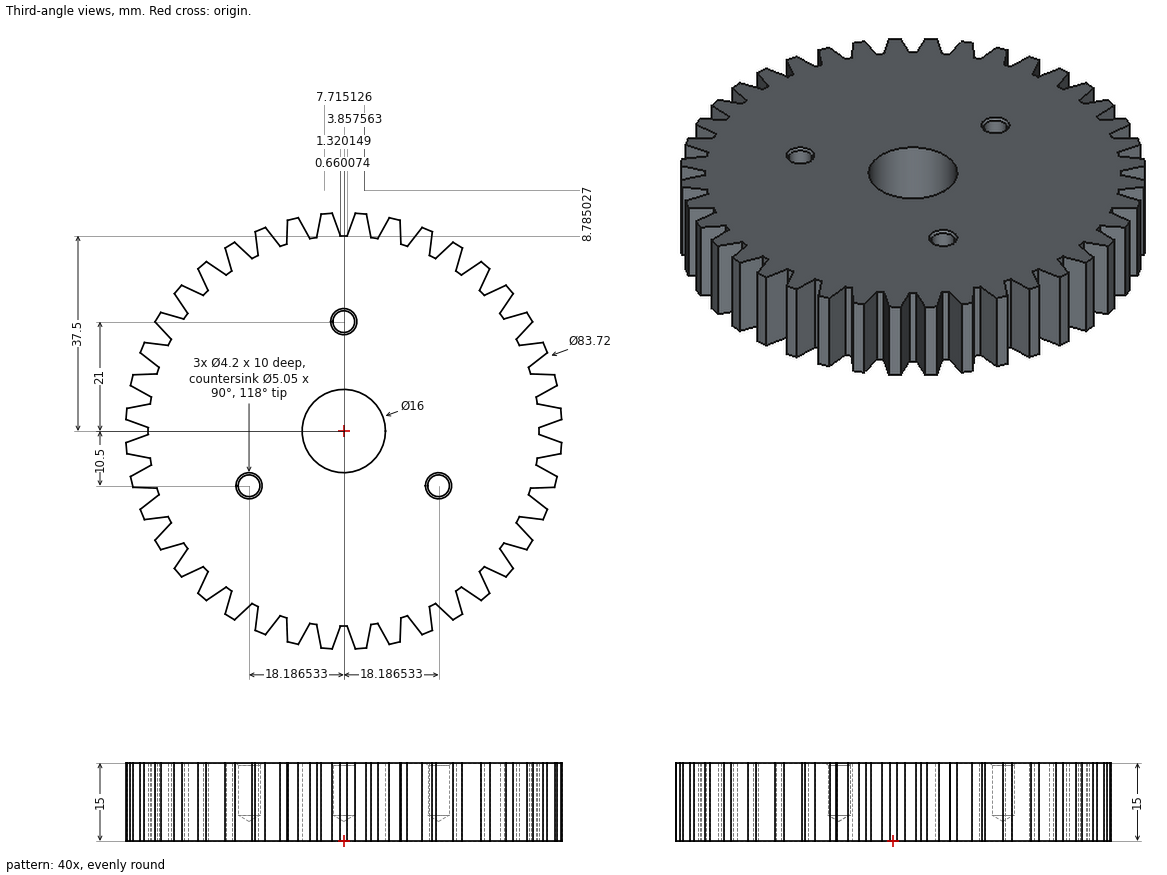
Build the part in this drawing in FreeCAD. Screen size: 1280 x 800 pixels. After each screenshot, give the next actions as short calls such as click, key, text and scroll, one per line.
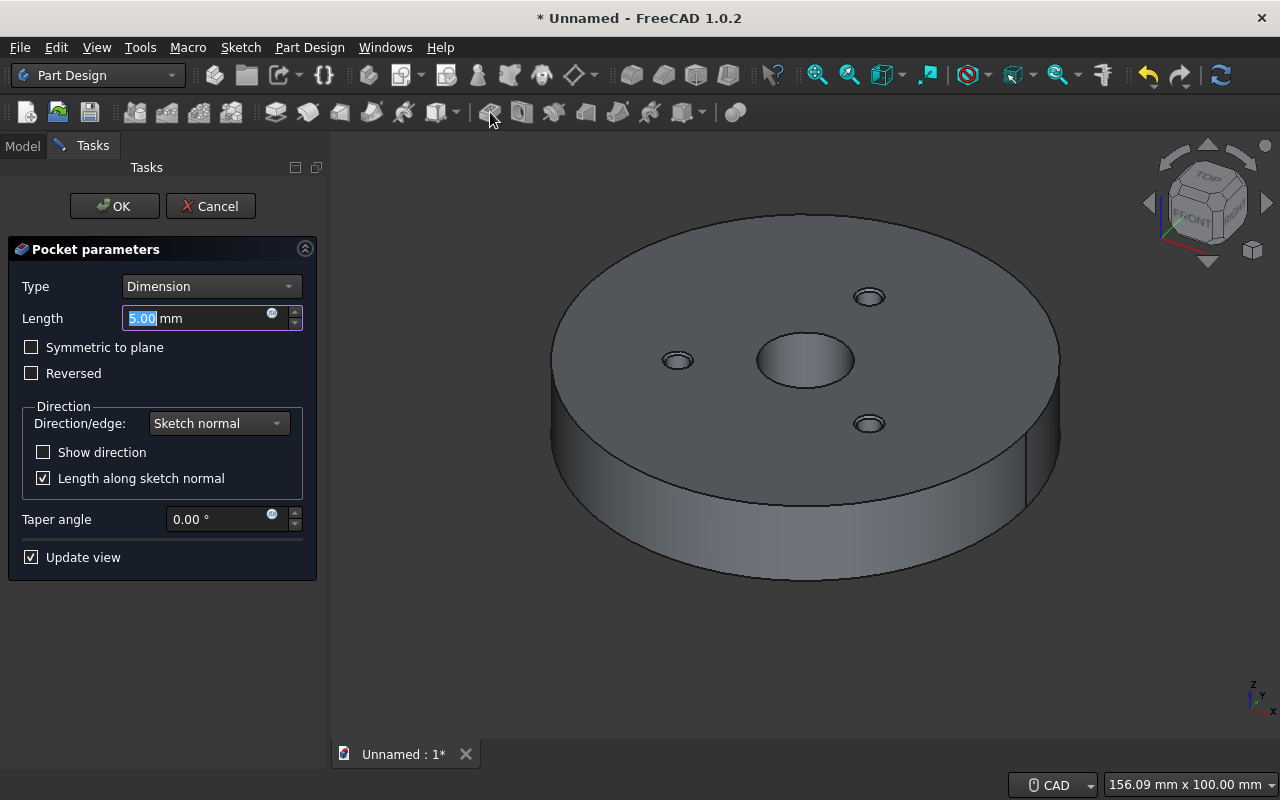
text(15)
key(Tab)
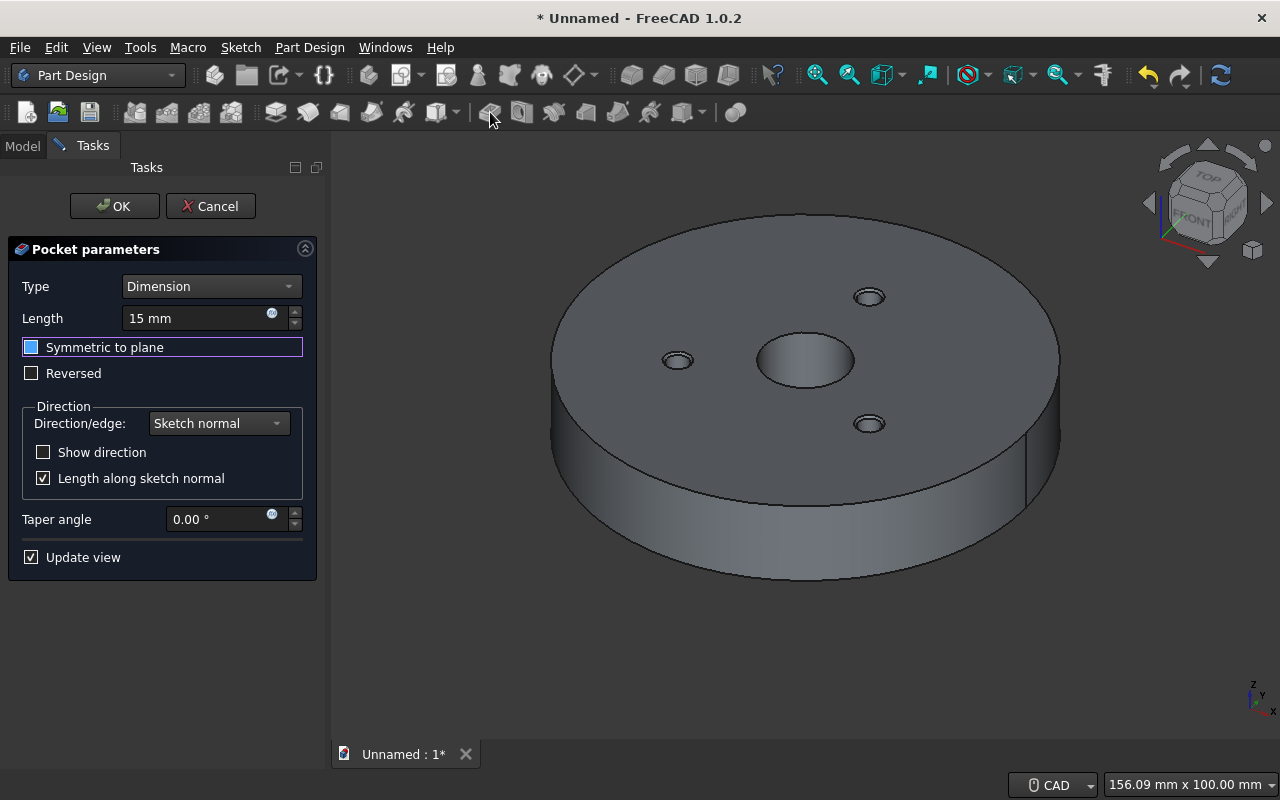
click(30, 373)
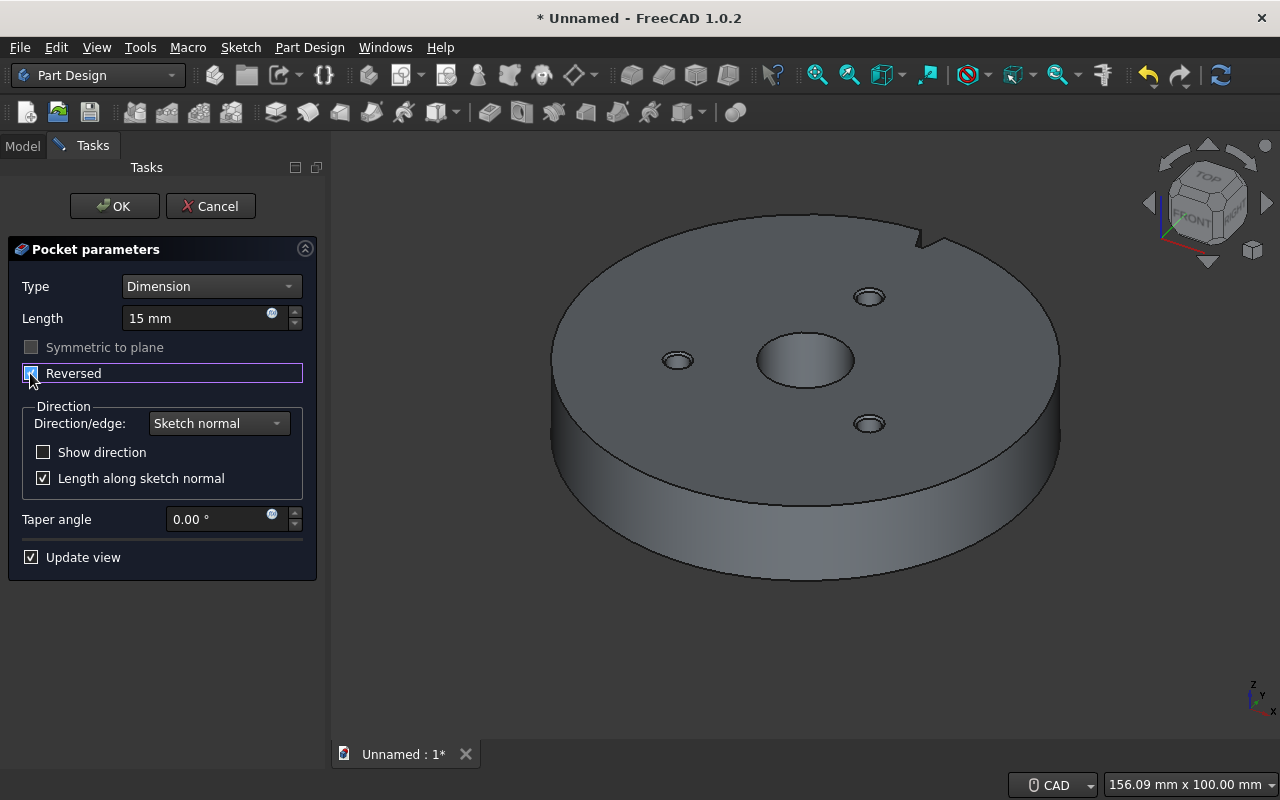
click(115, 206)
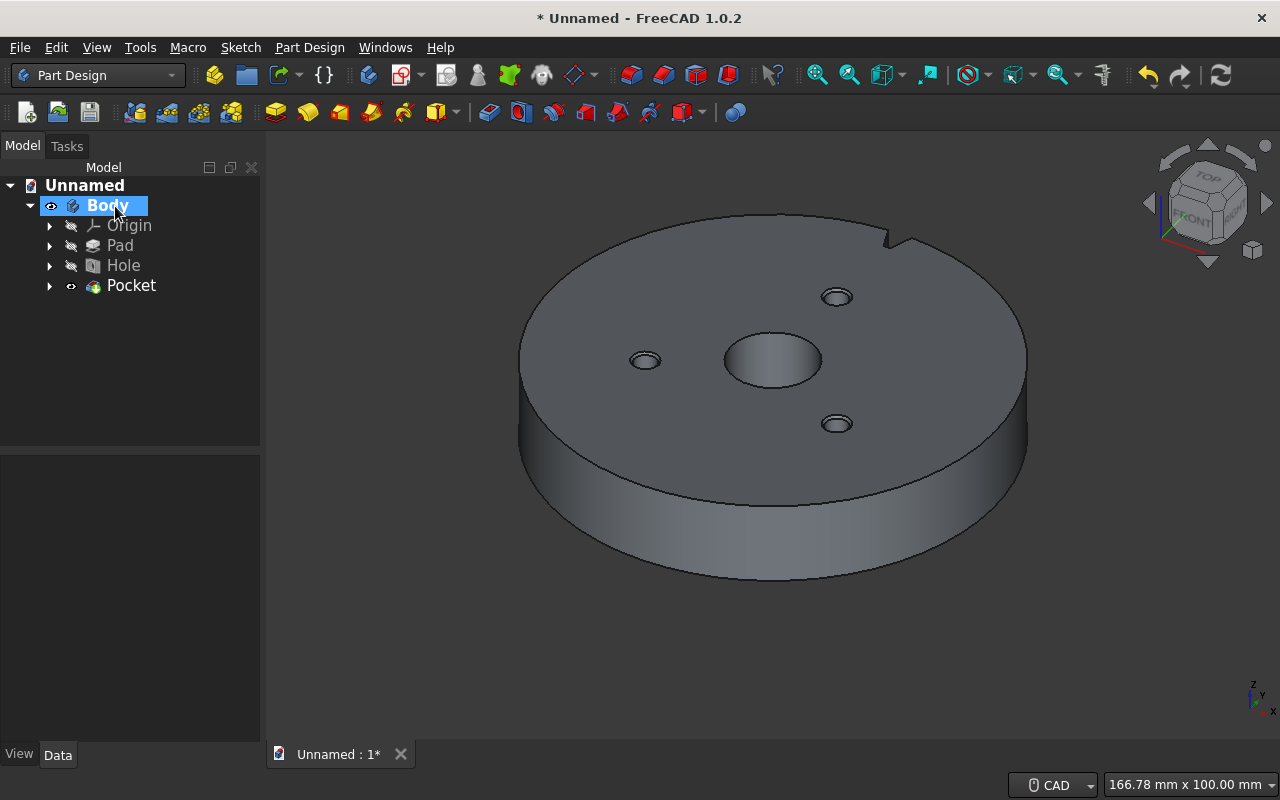
click(116, 286)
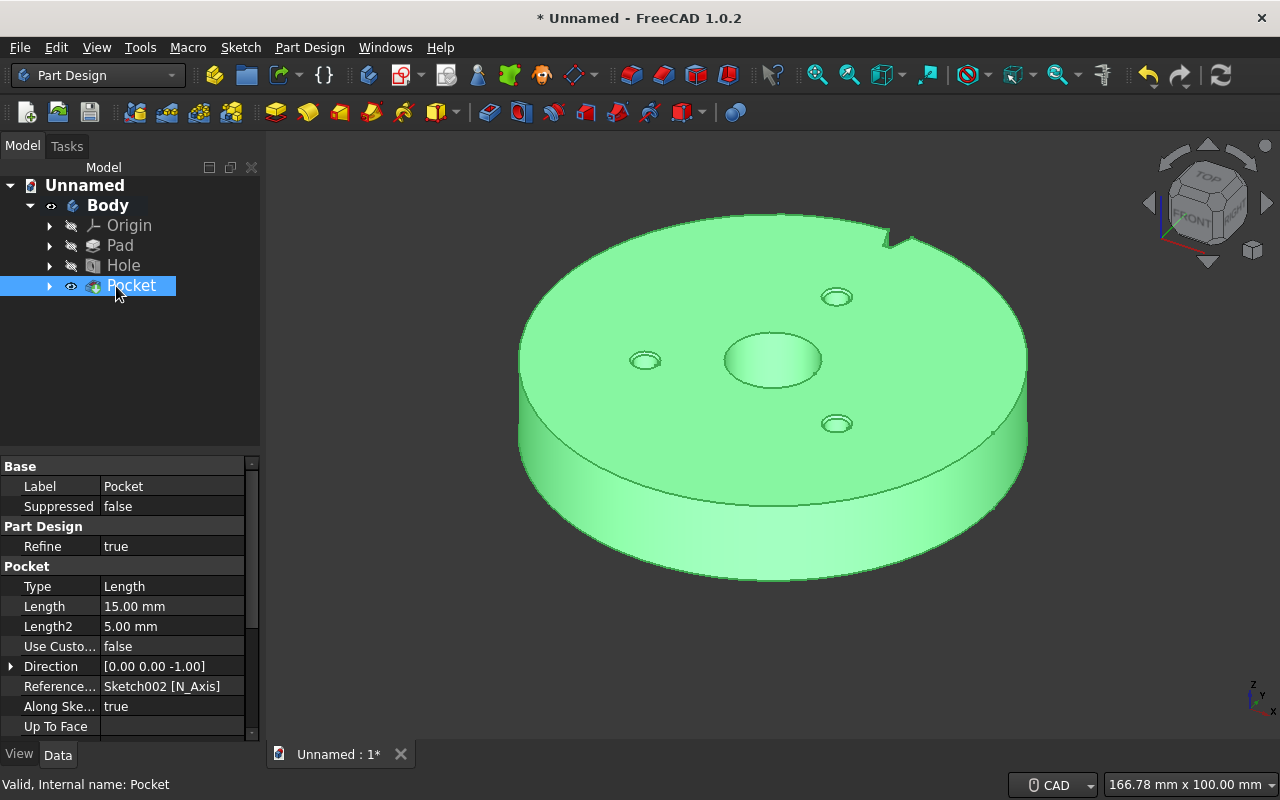
click(200, 112)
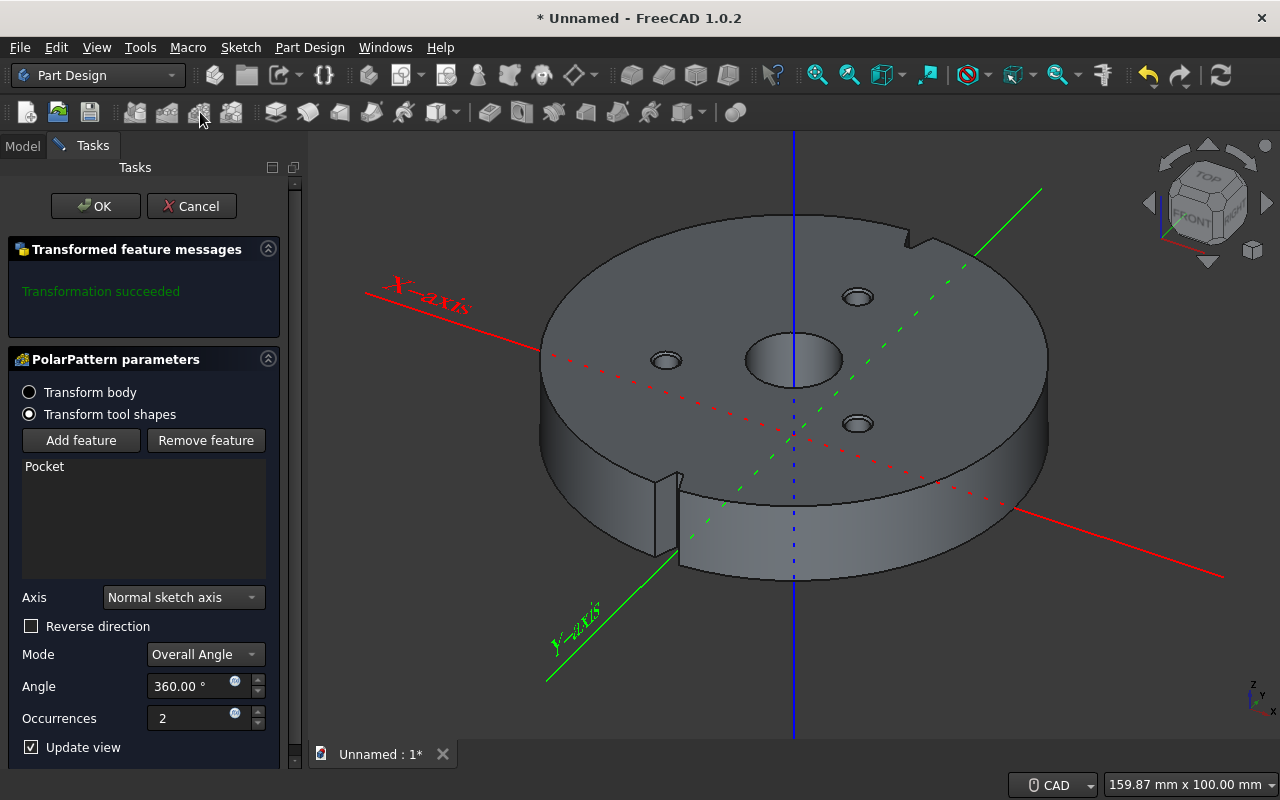
click(184, 598)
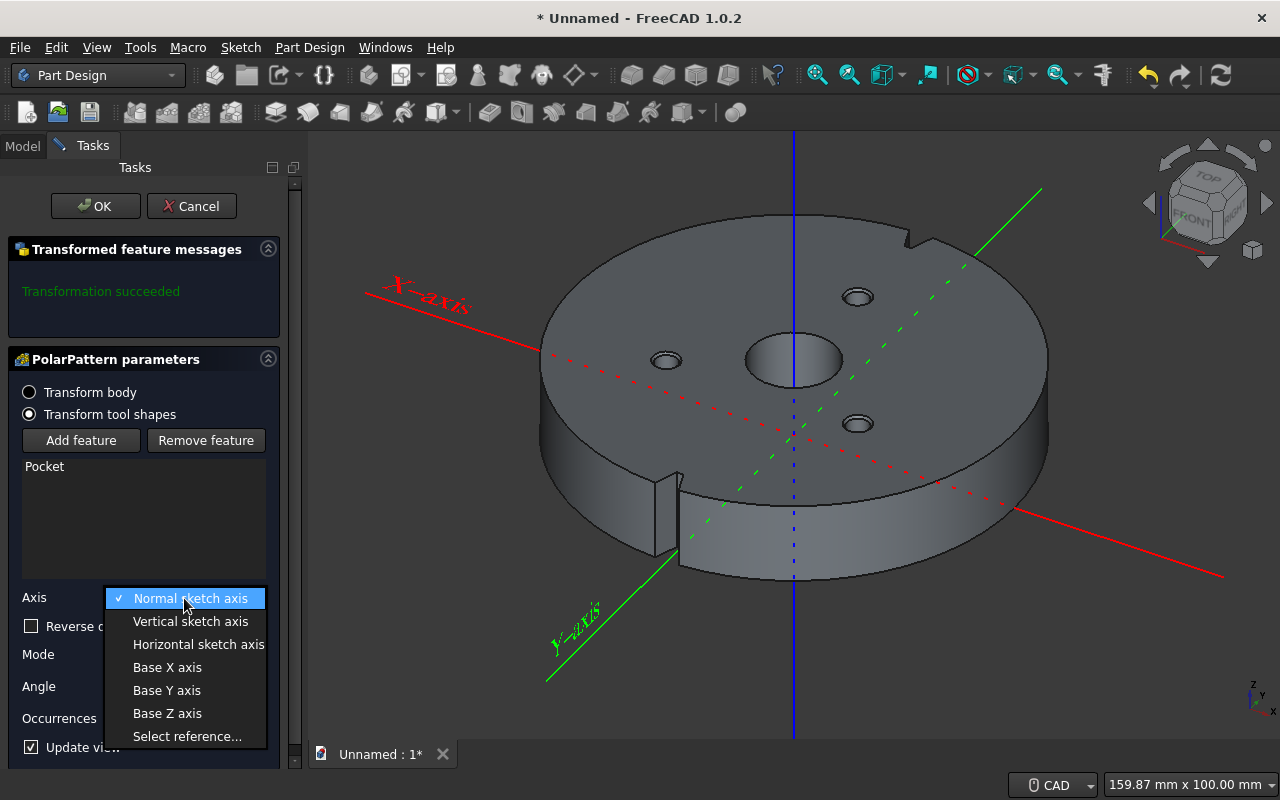
click(184, 714)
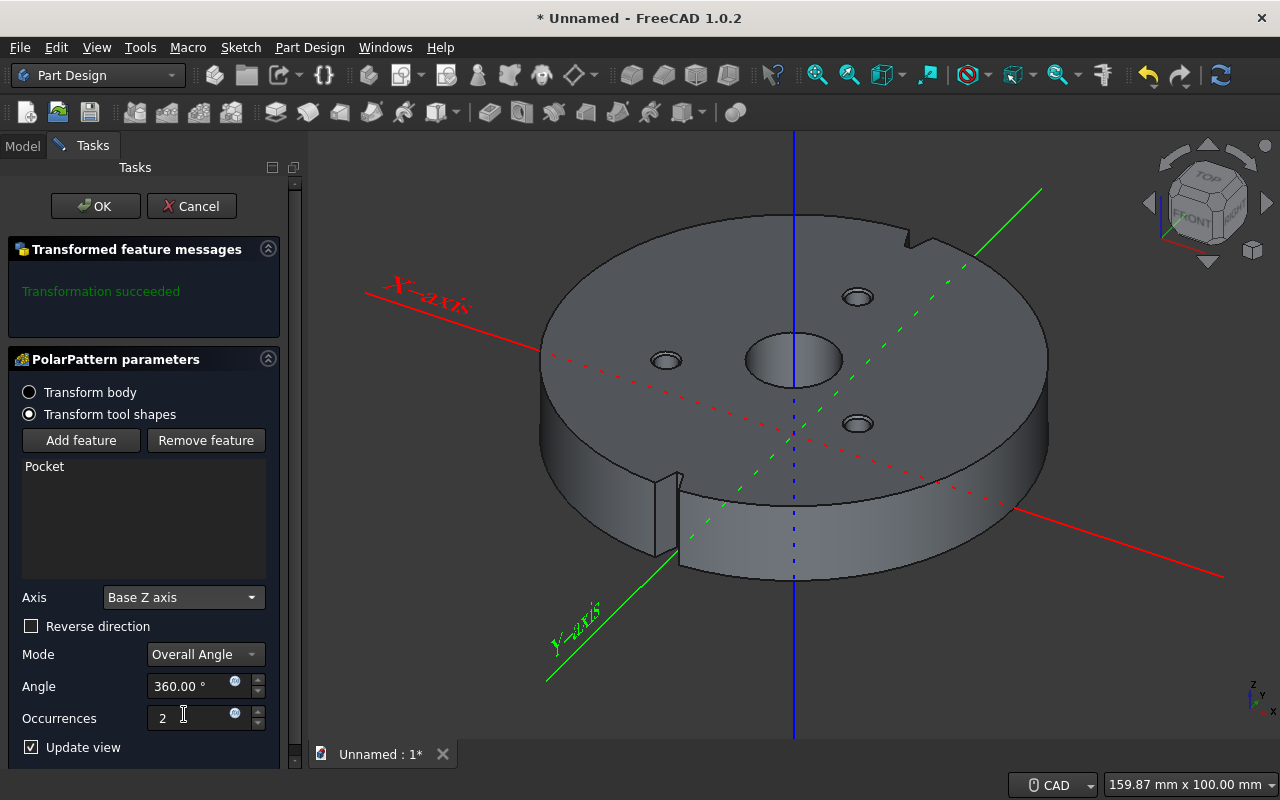
triple_click(198, 718)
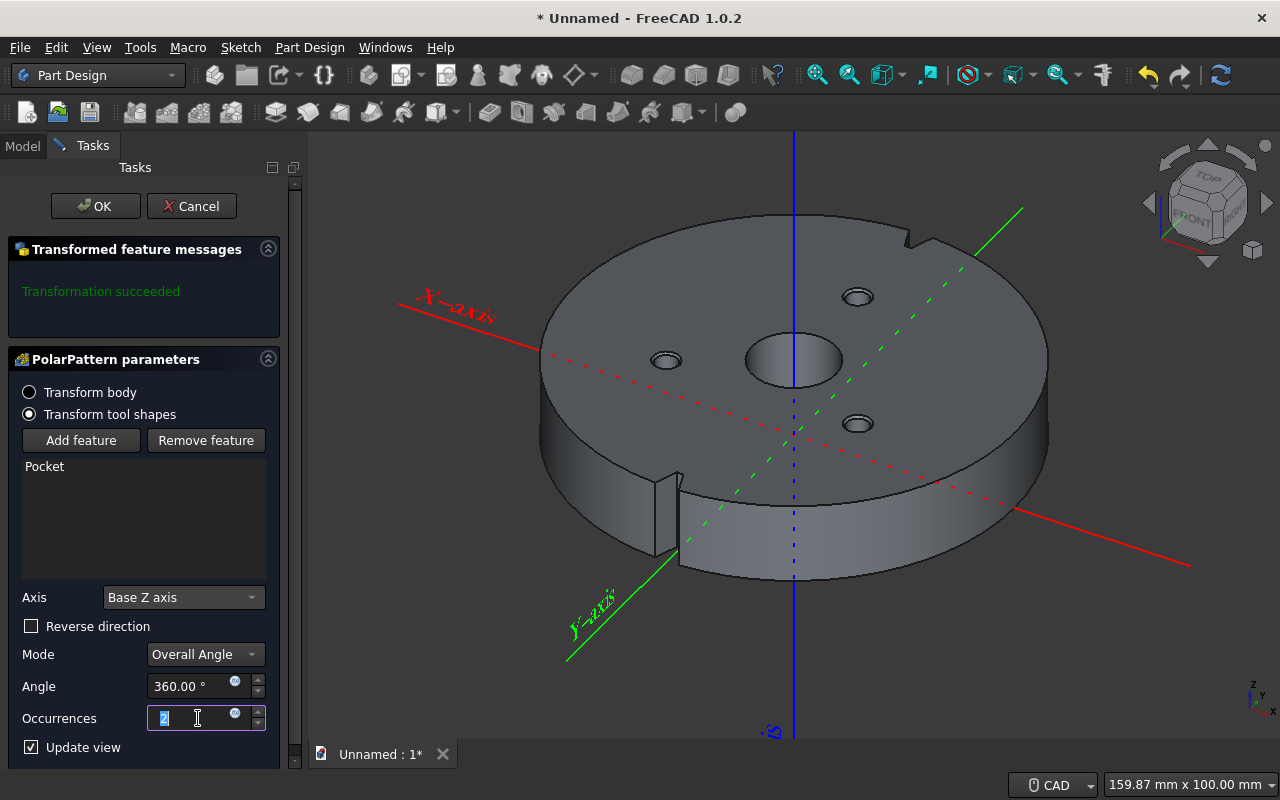
text(40)
key(Tab)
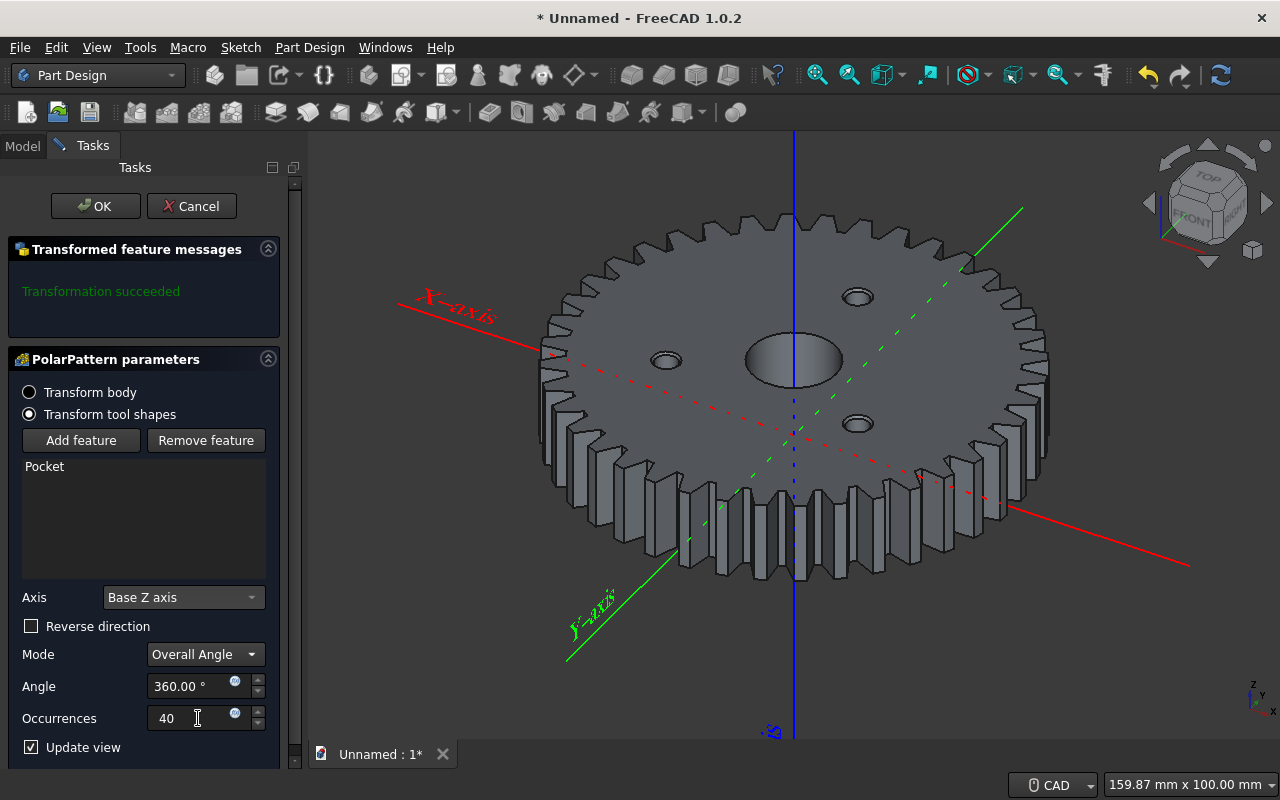
click(96, 206)